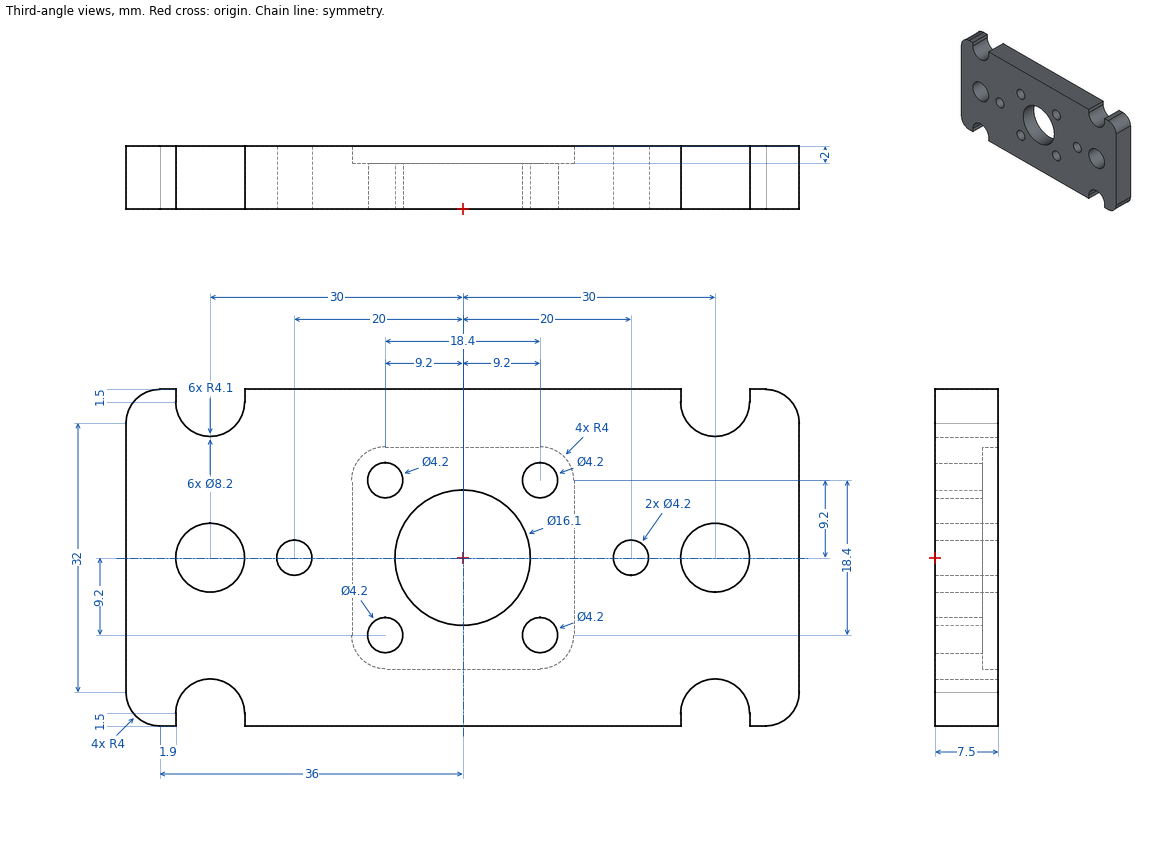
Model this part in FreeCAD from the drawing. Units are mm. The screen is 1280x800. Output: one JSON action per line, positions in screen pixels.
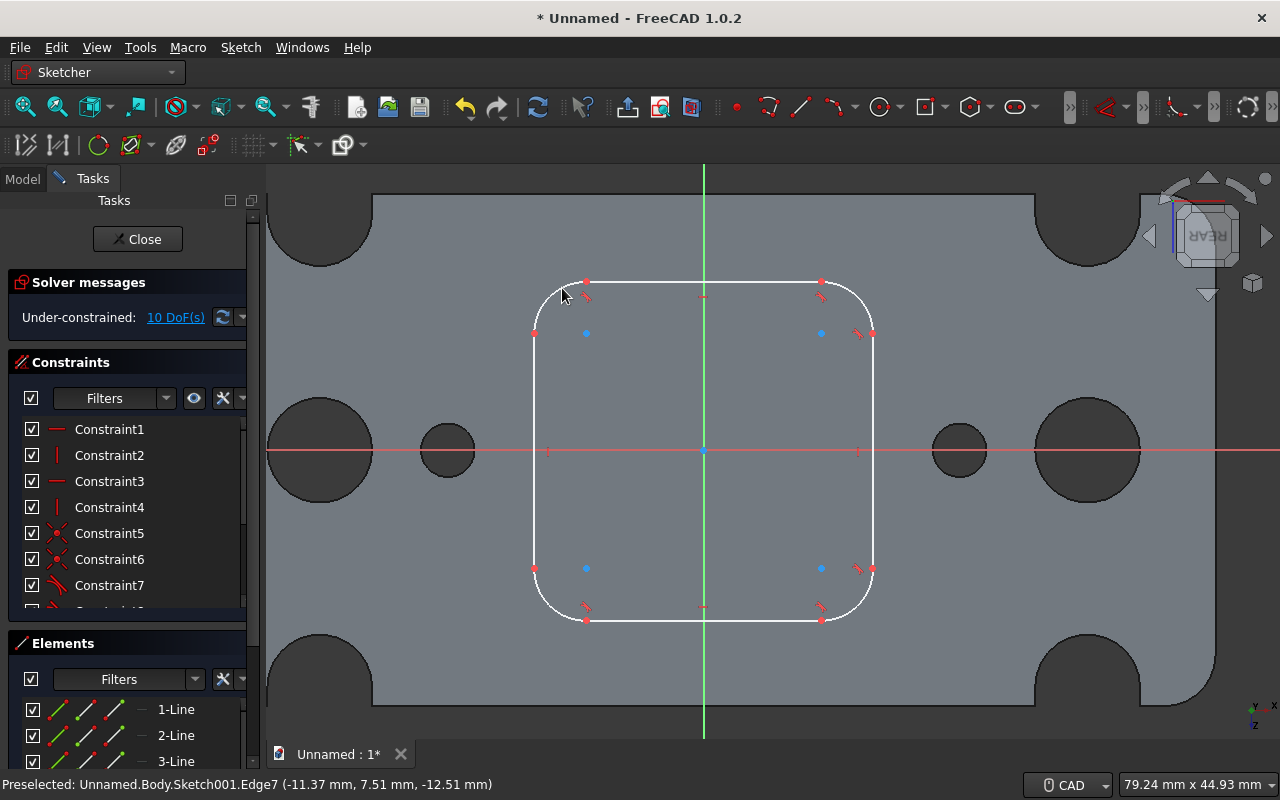
{"action": "left_click", "coordinate": [534, 404]}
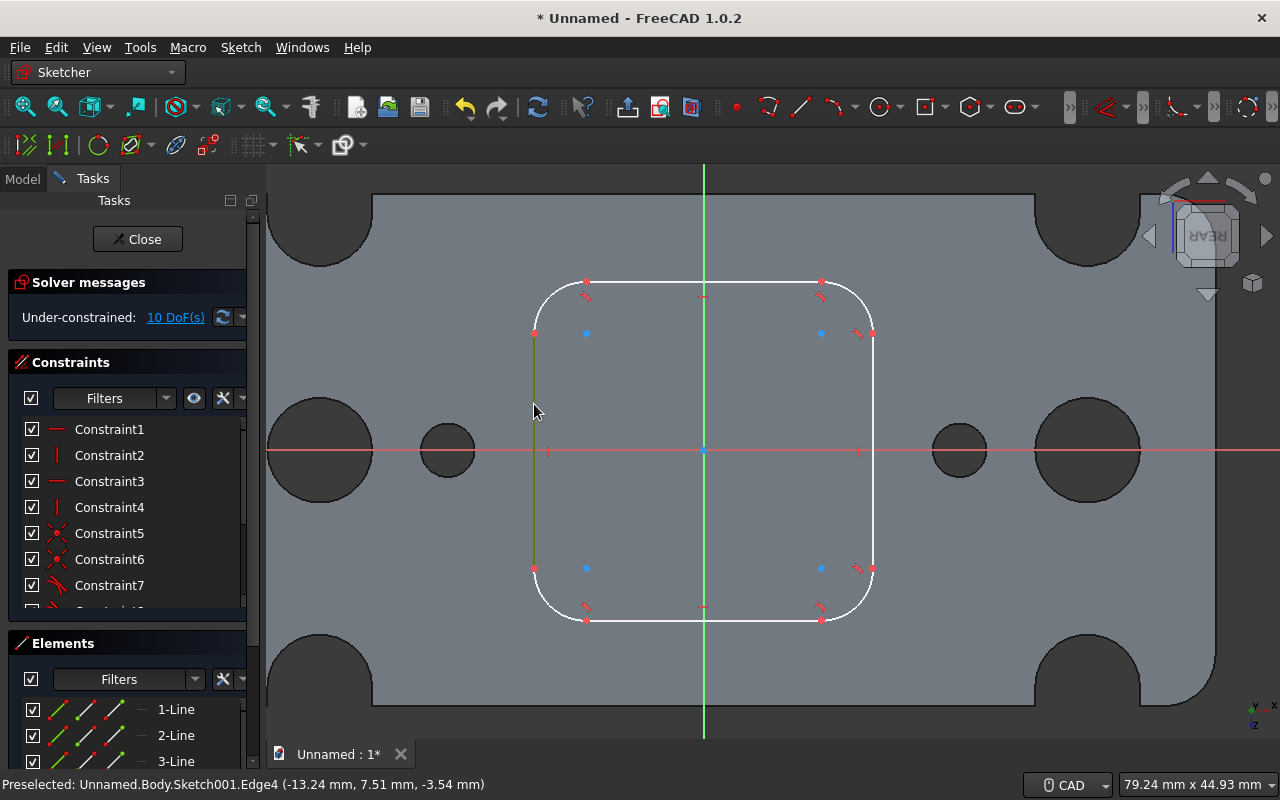
{"action": "left_click", "coordinate": [563, 288]}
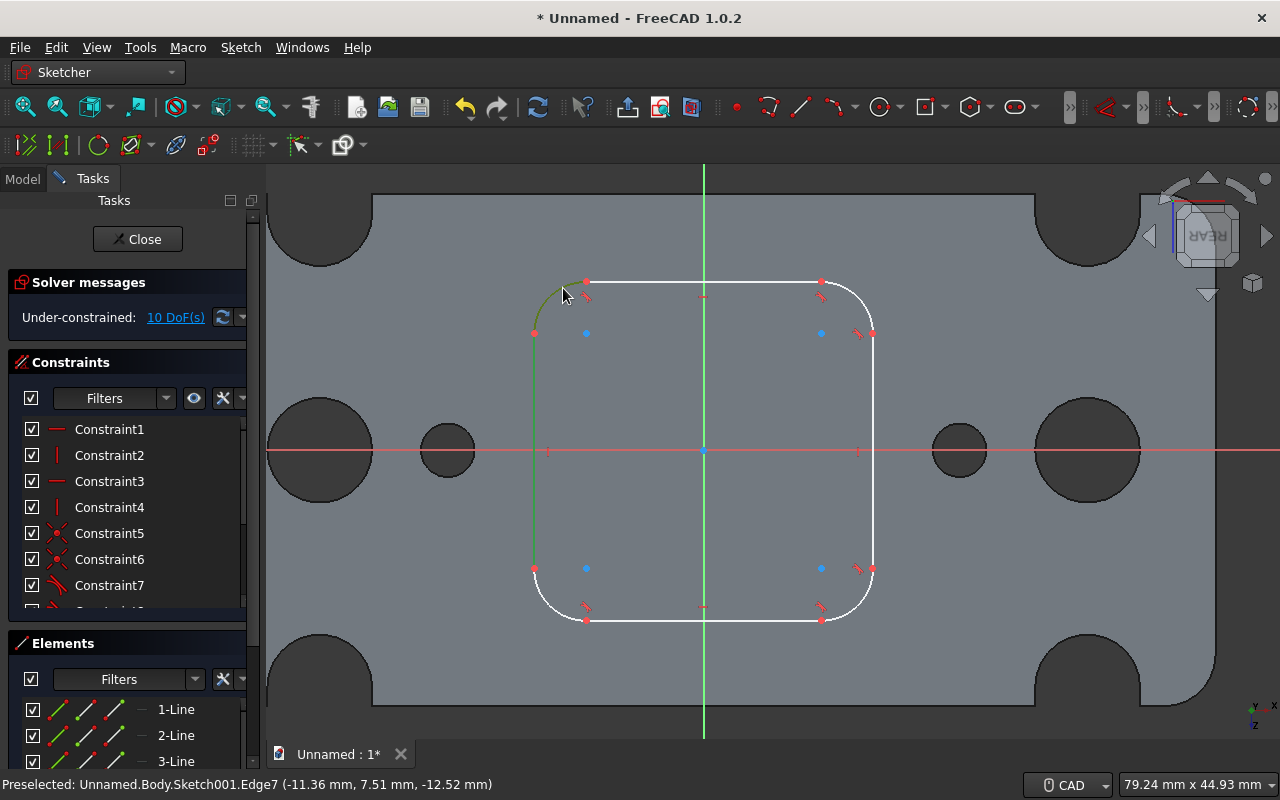
{"action": "key", "text": "t"}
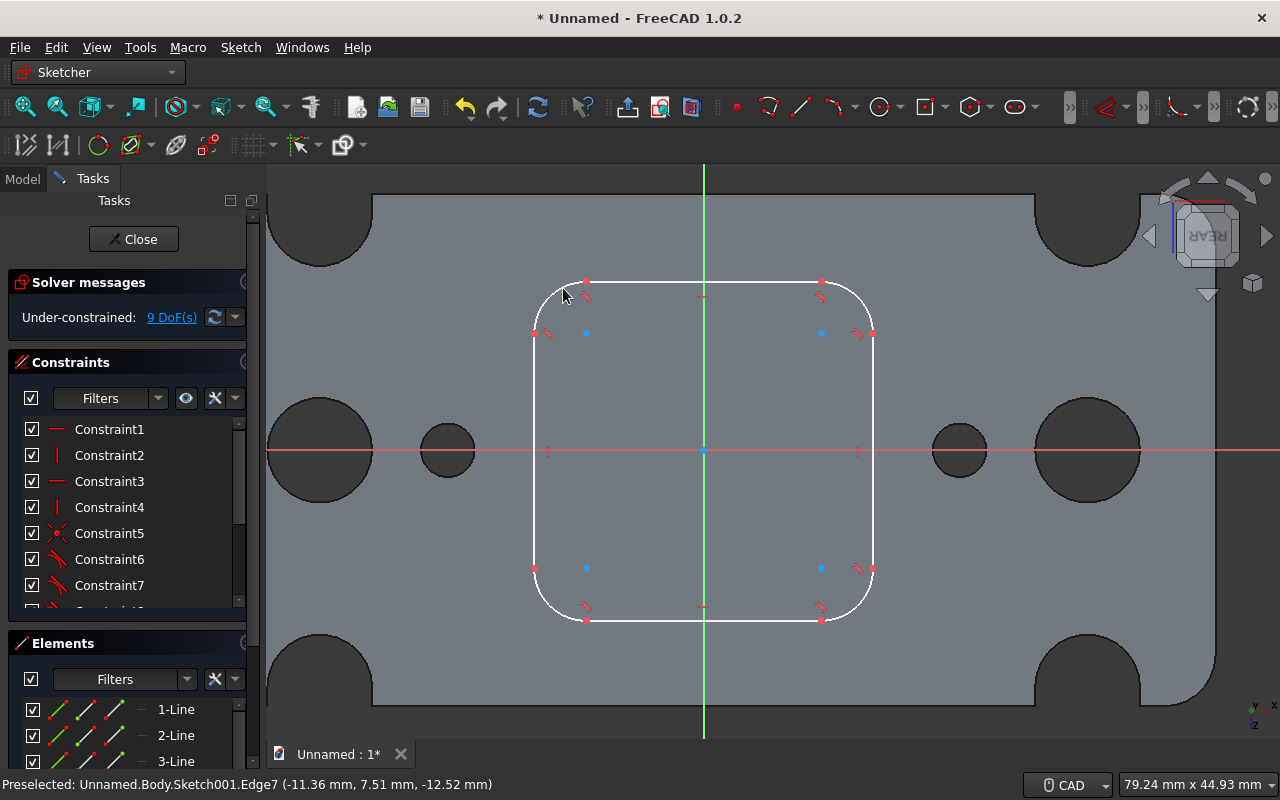
{"action": "left_click", "coordinate": [534, 404]}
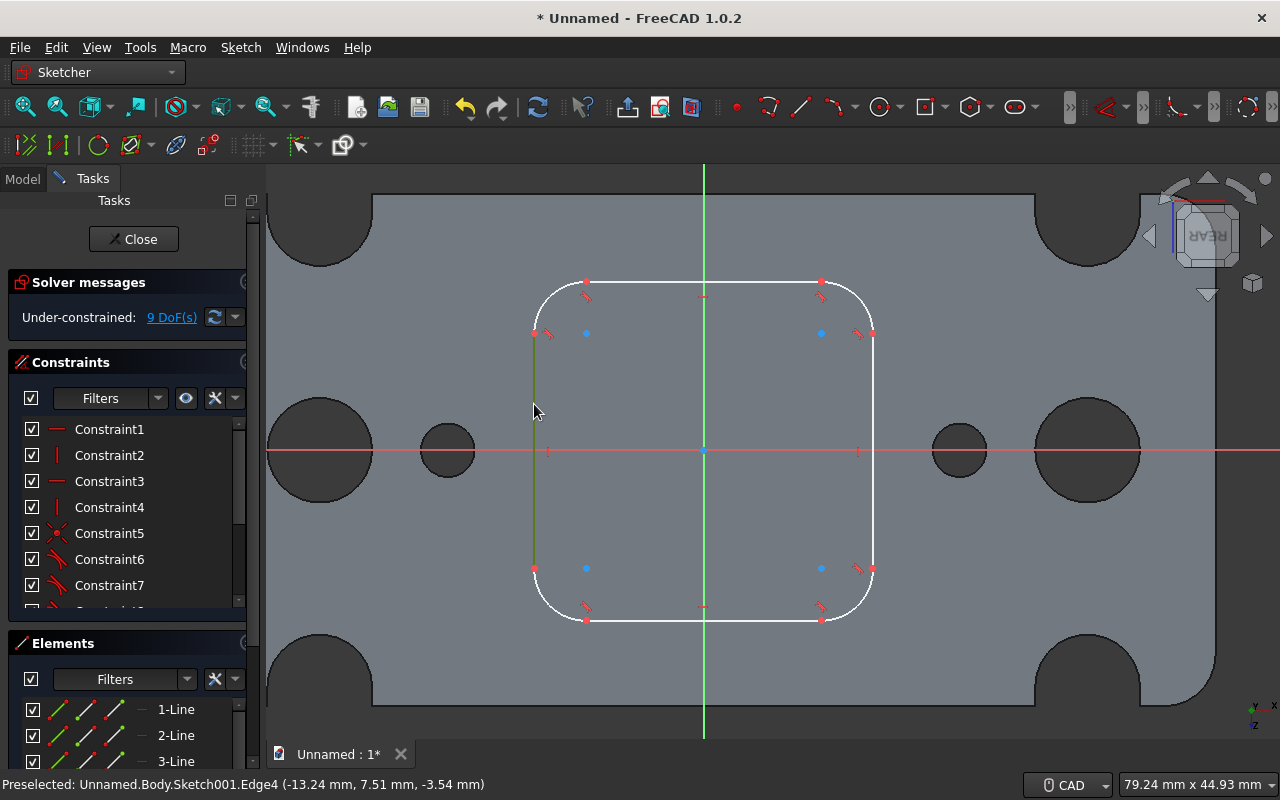
{"action": "left_click", "coordinate": [540, 593]}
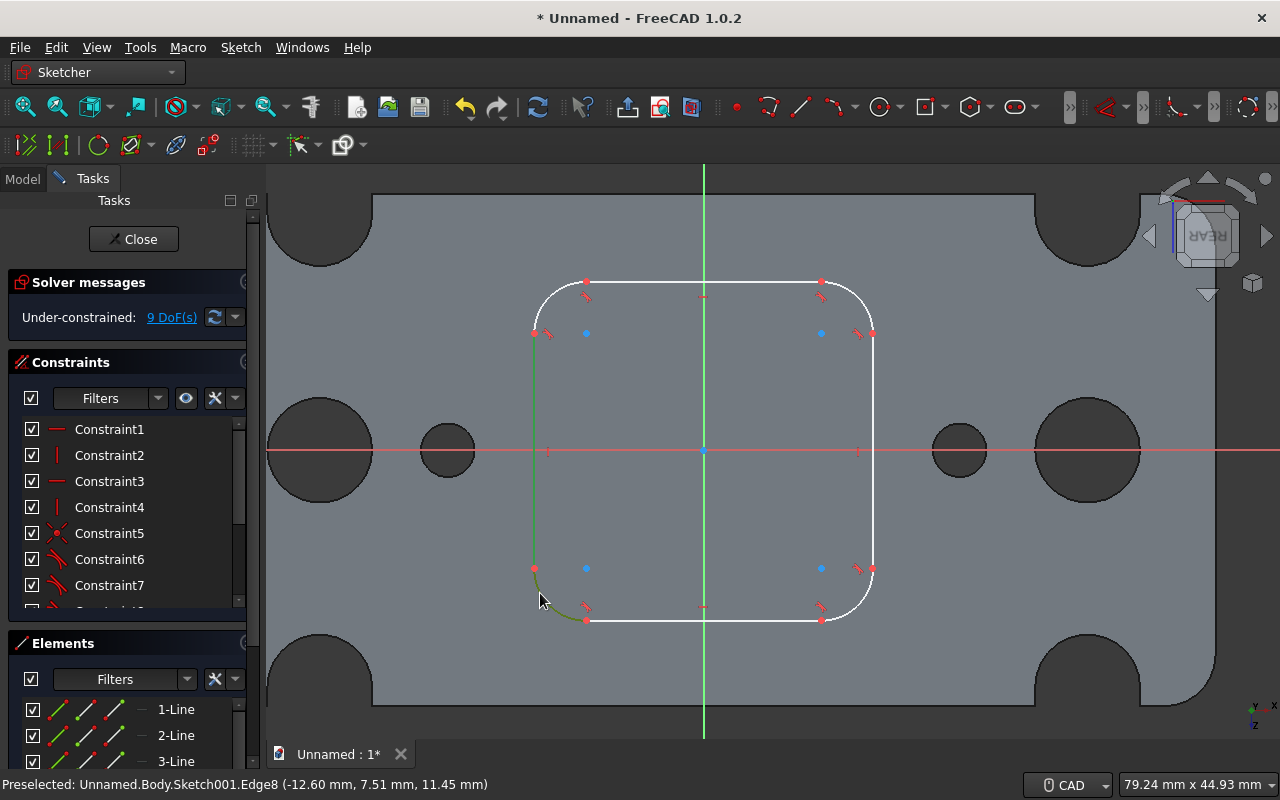
{"action": "key", "text": "t"}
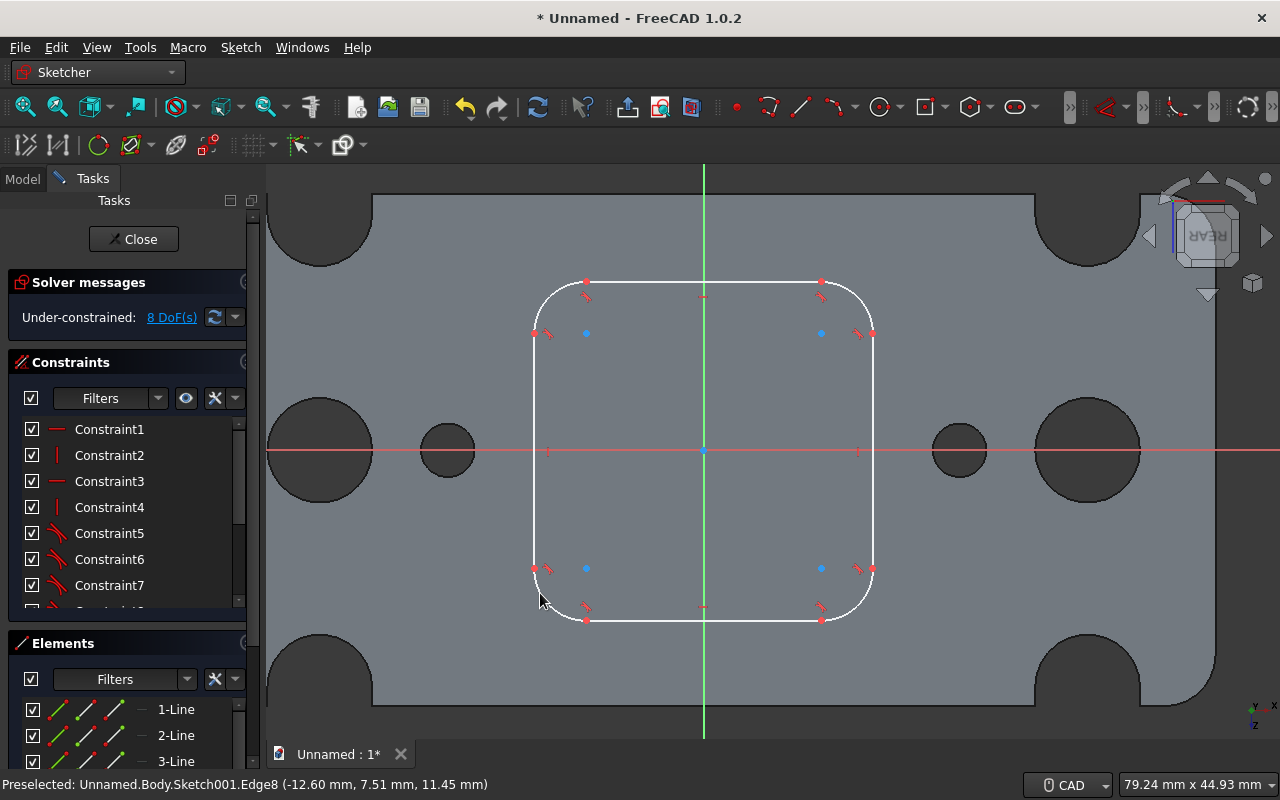
{"action": "left_click", "coordinate": [845, 615]}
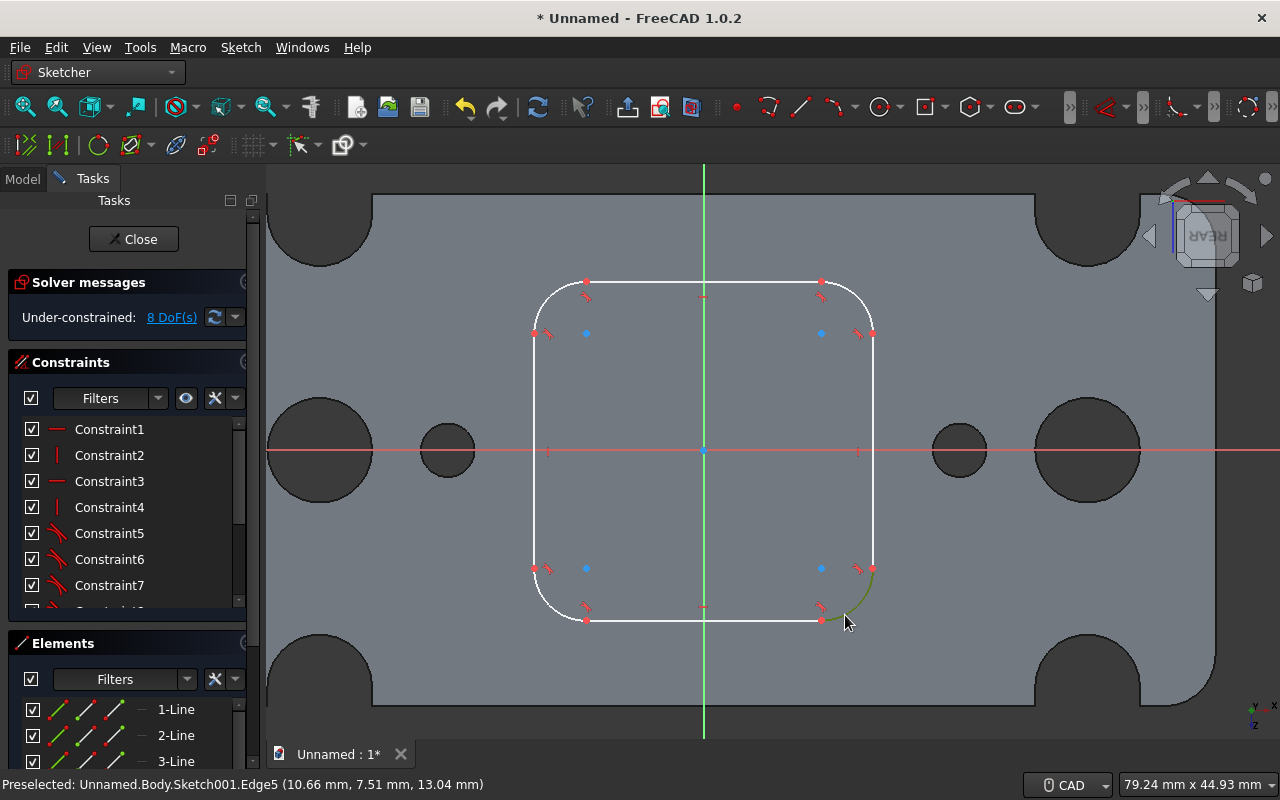
{"action": "left_click", "coordinate": [867, 310]}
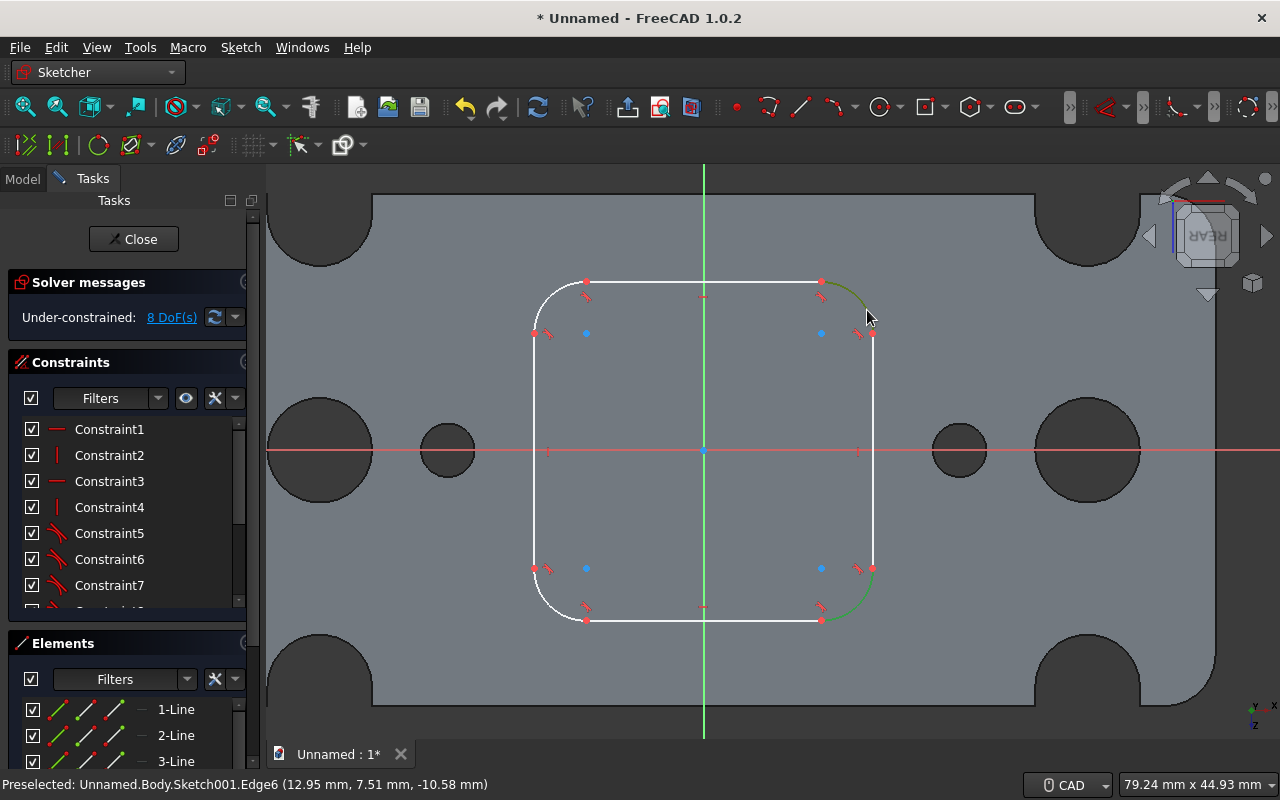
{"action": "left_click", "coordinate": [563, 288]}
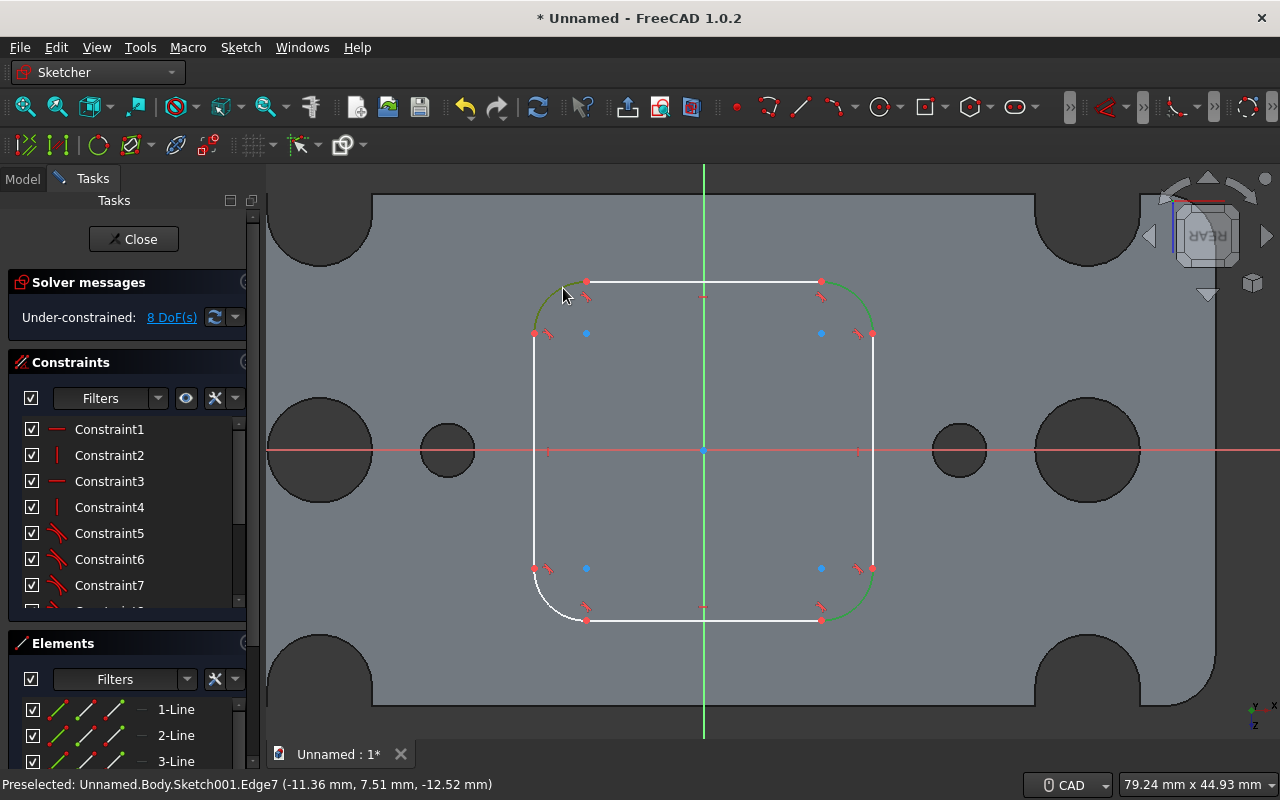
{"action": "left_click", "coordinate": [540, 592]}